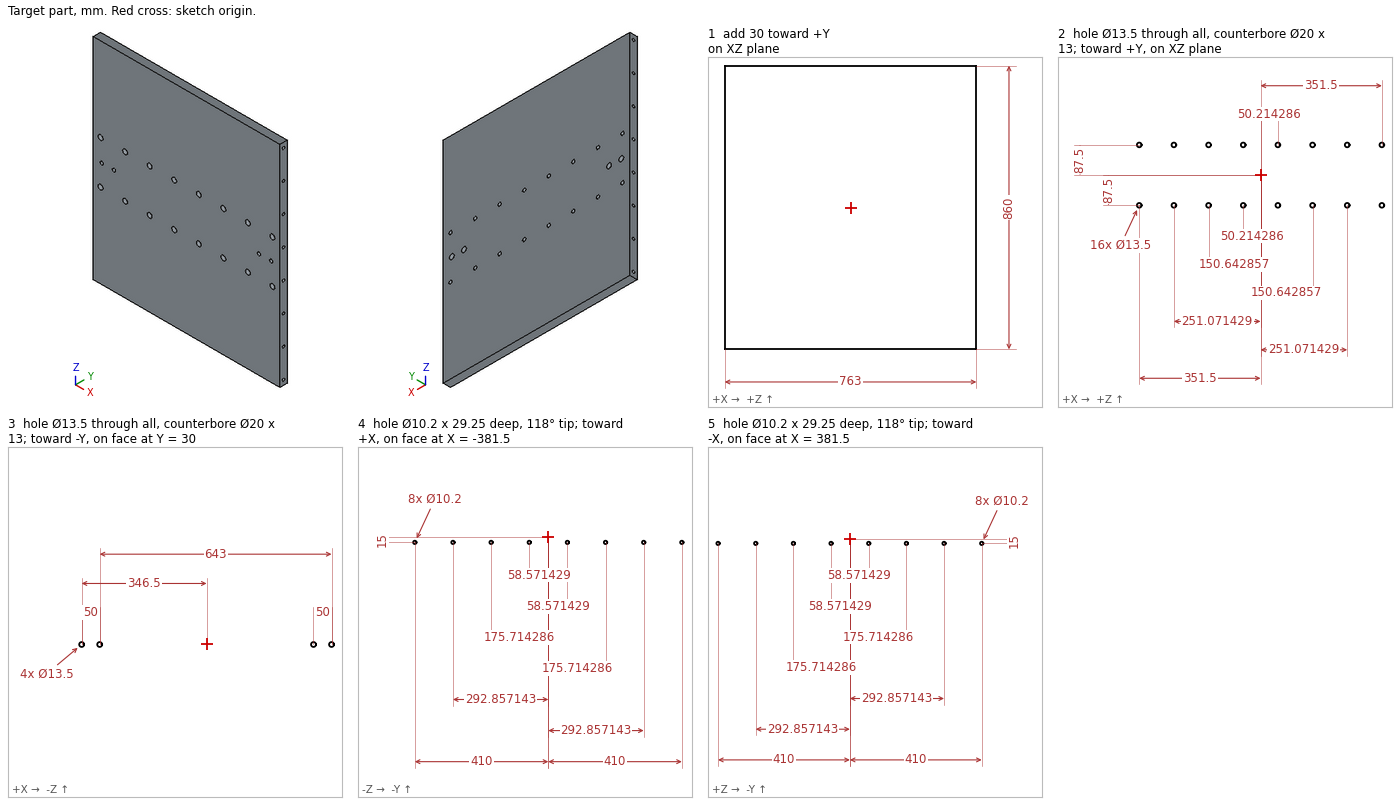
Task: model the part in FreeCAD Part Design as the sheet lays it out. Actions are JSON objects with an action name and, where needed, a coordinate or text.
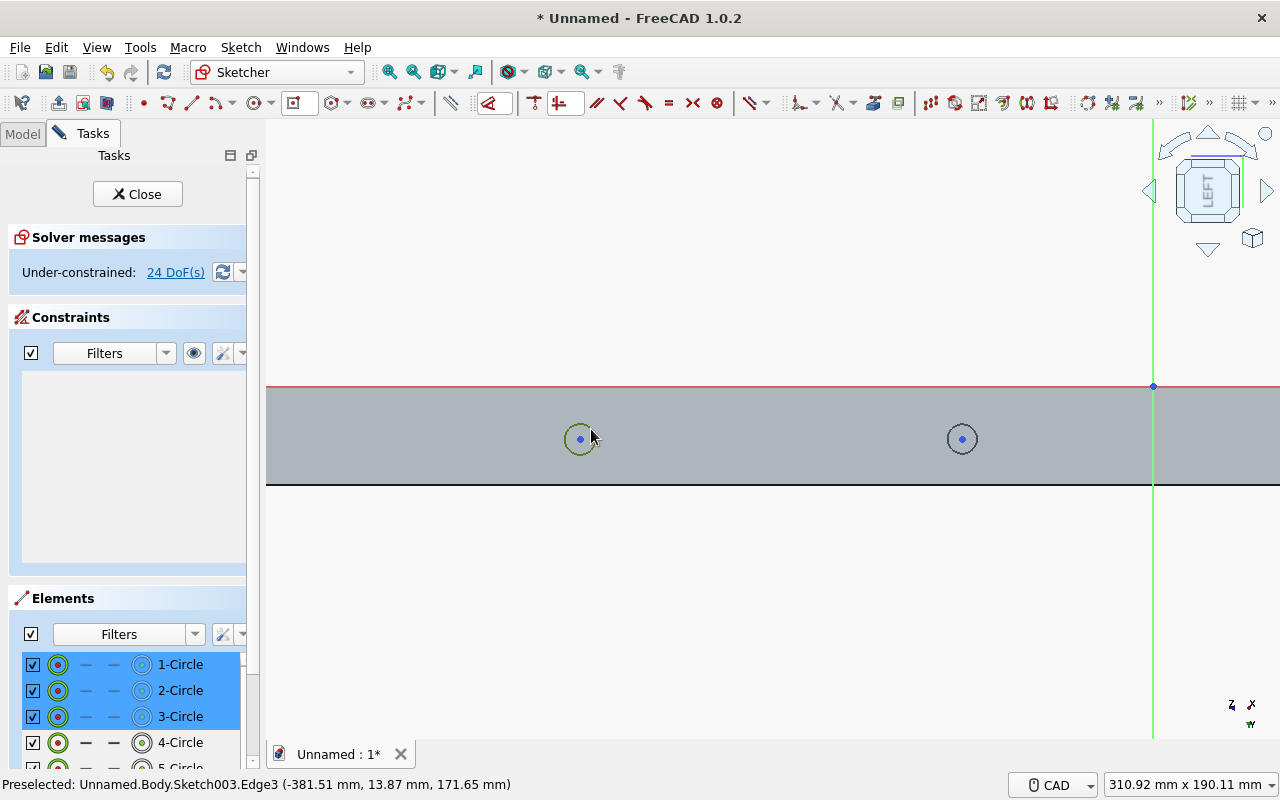
{"action": "left_click", "coordinate": [973, 429]}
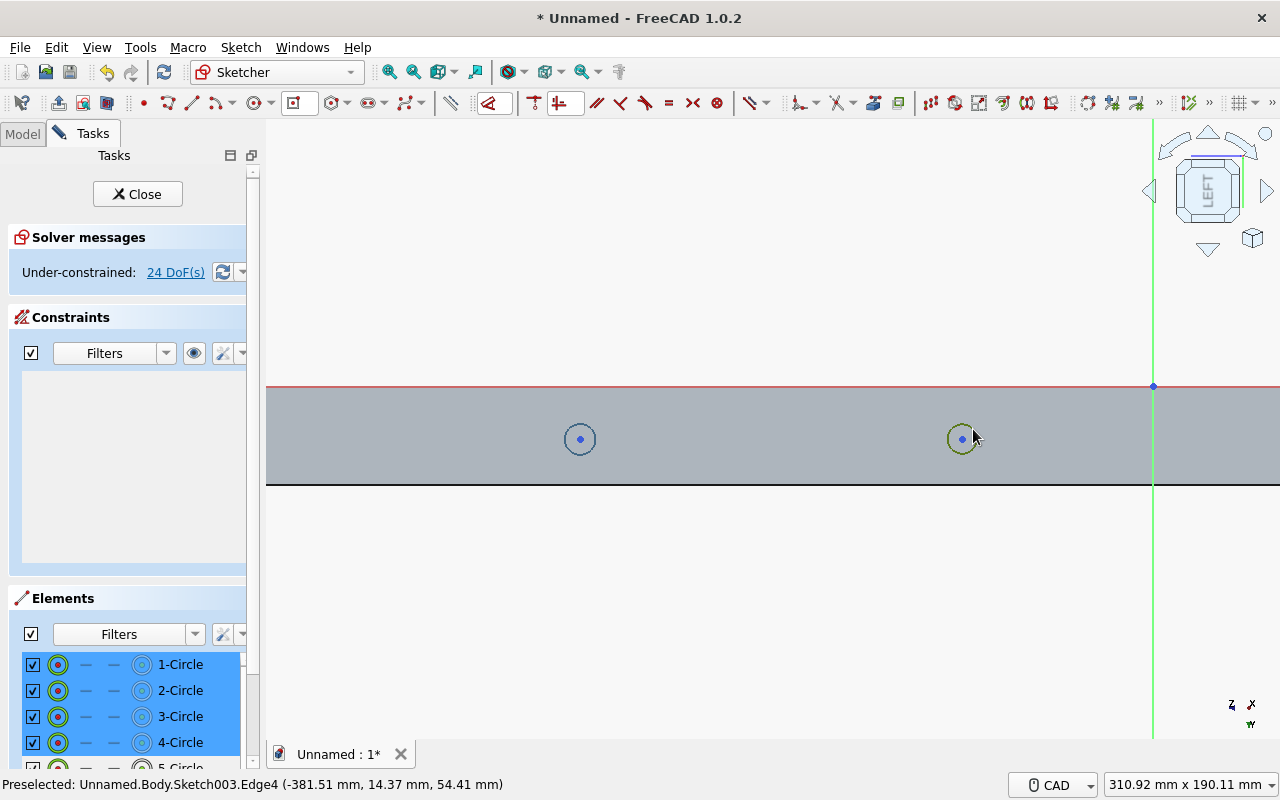
{"action": "scroll", "coordinate": [591, 431], "scroll_direction": "down", "scroll_amount": 8}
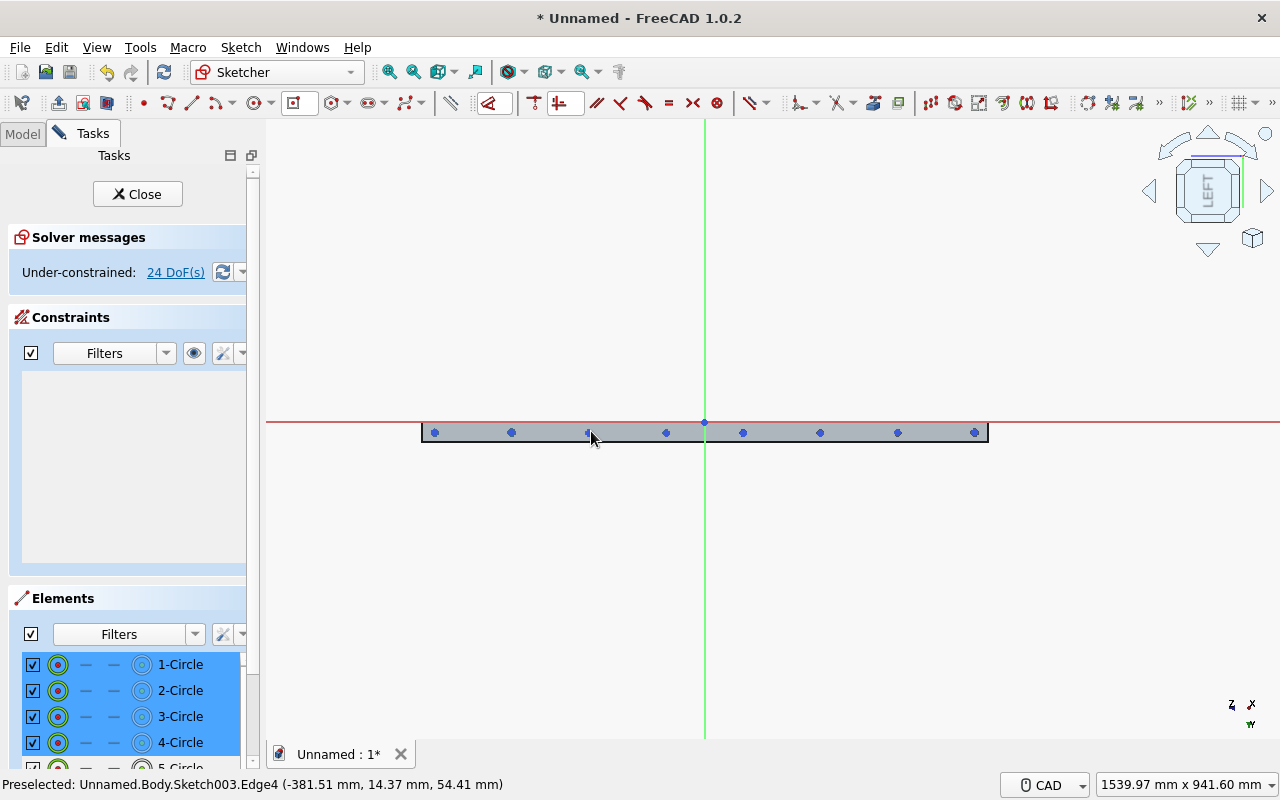
{"action": "scroll", "coordinate": [745, 431], "scroll_direction": "up", "scroll_amount": 8}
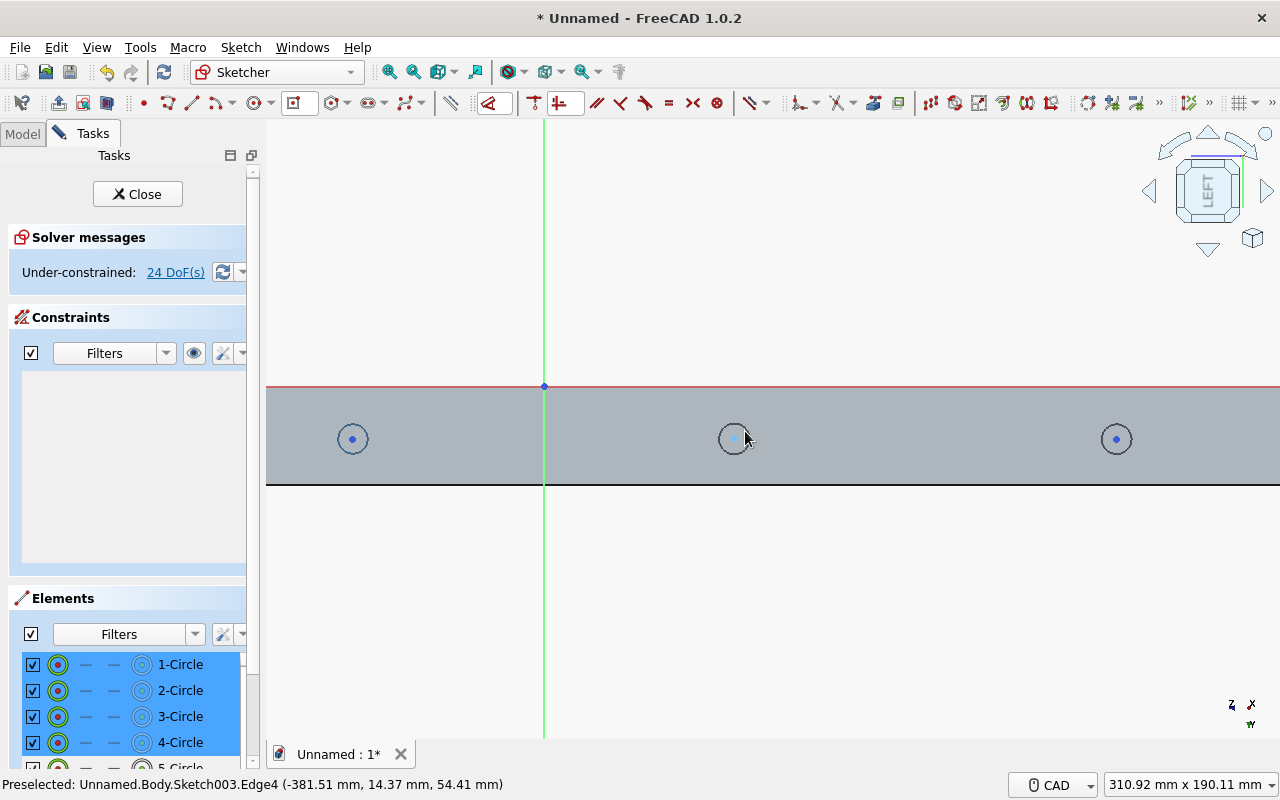
{"action": "left_click", "coordinate": [745, 428]}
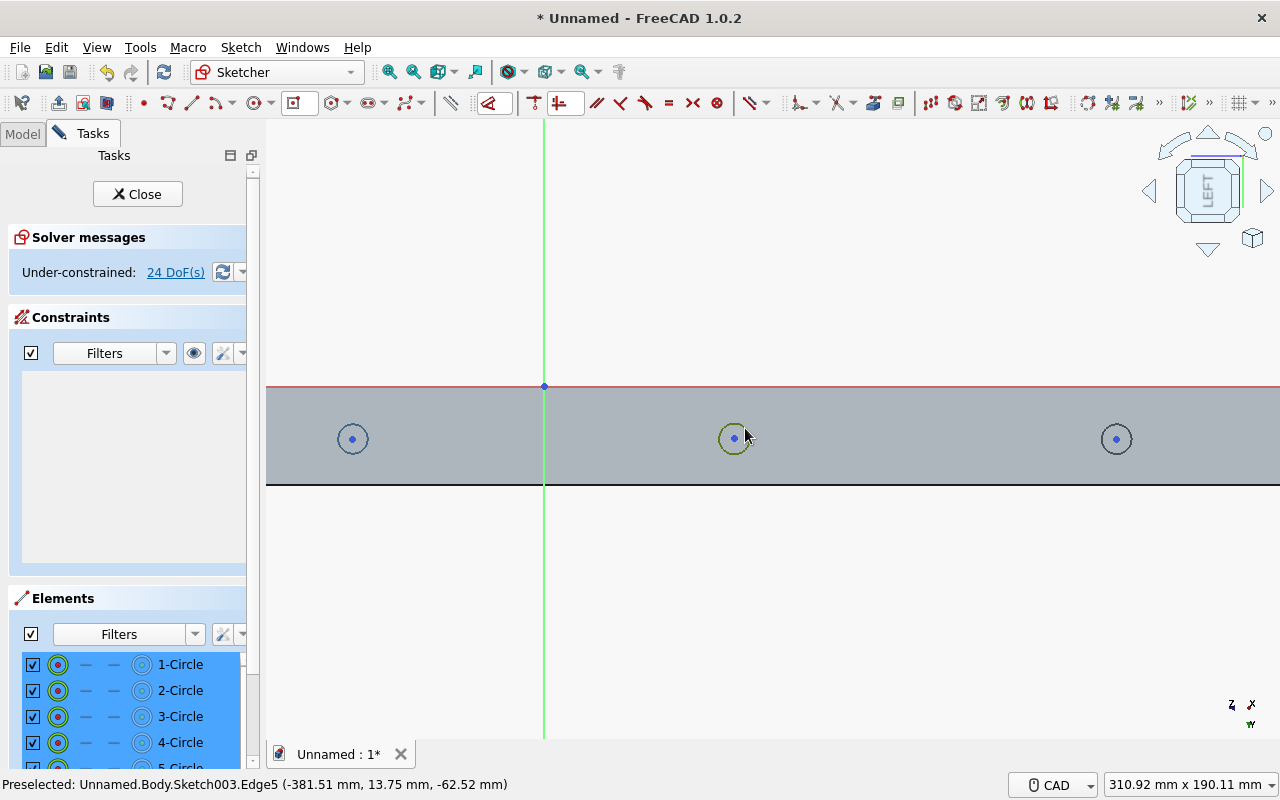
{"action": "left_click", "coordinate": [1106, 429]}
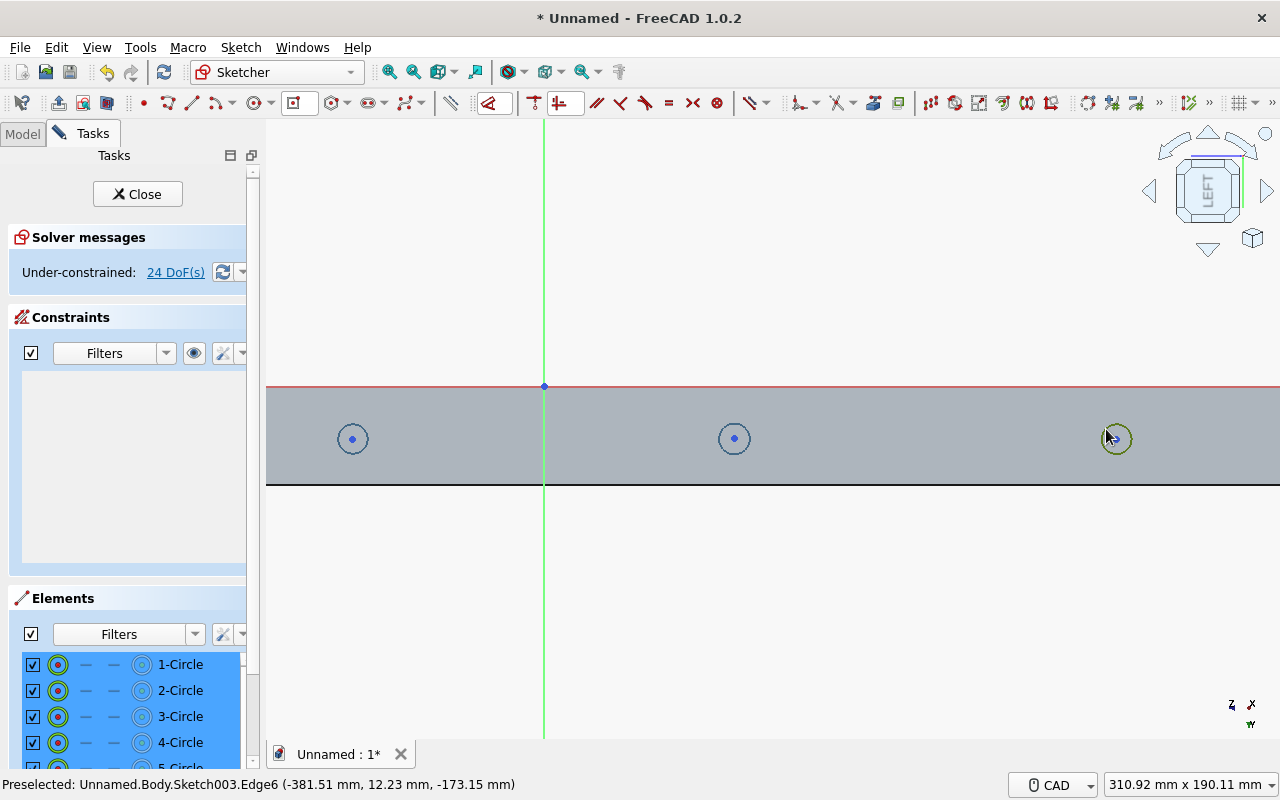
{"action": "scroll", "coordinate": [745, 431], "scroll_direction": "down", "scroll_amount": 8}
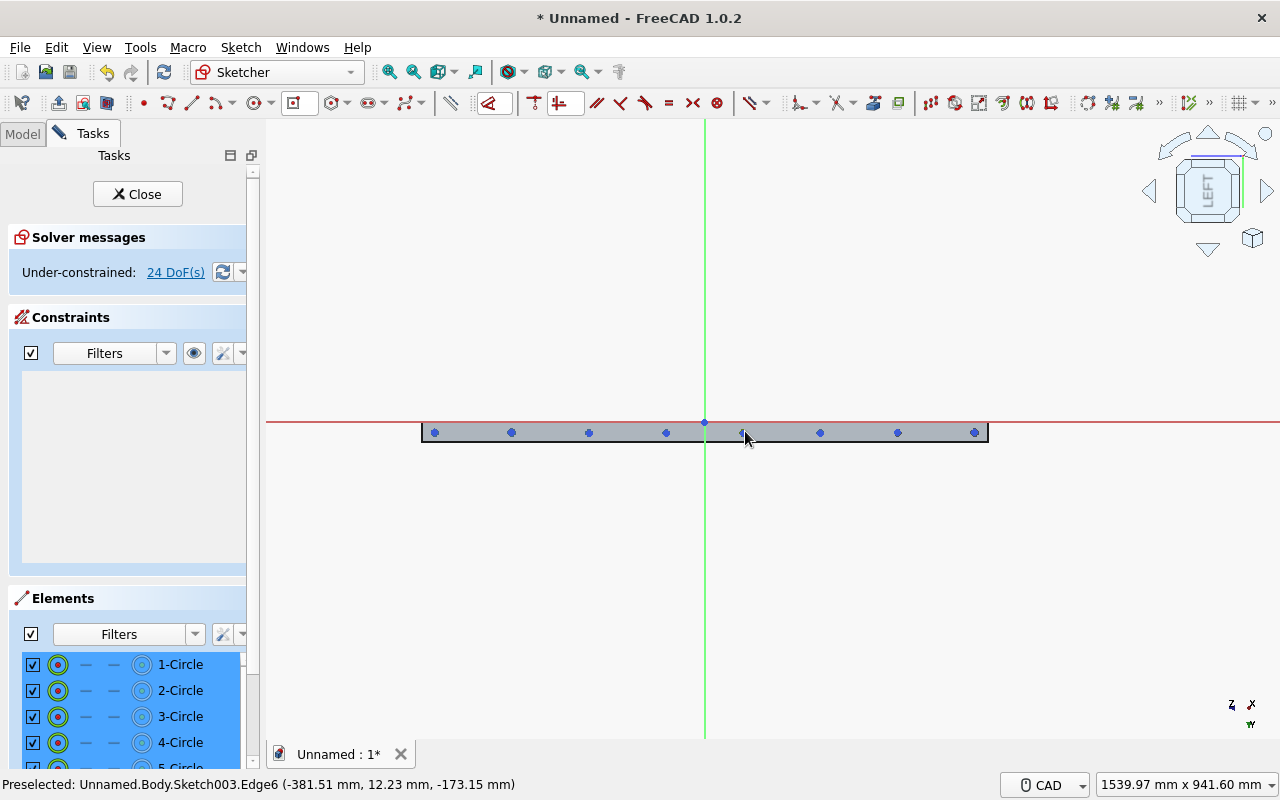
{"action": "scroll", "coordinate": [900, 431], "scroll_direction": "up", "scroll_amount": 8}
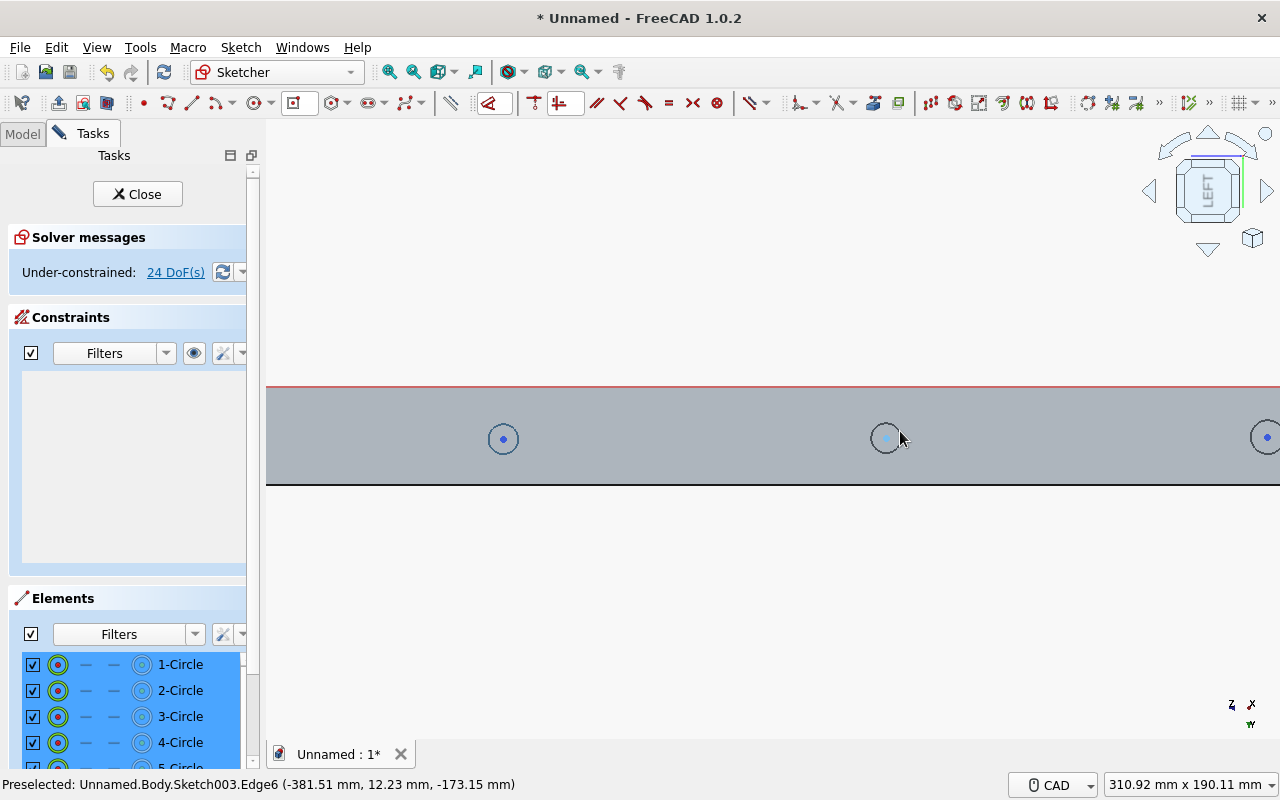
{"action": "left_click", "coordinate": [897, 428]}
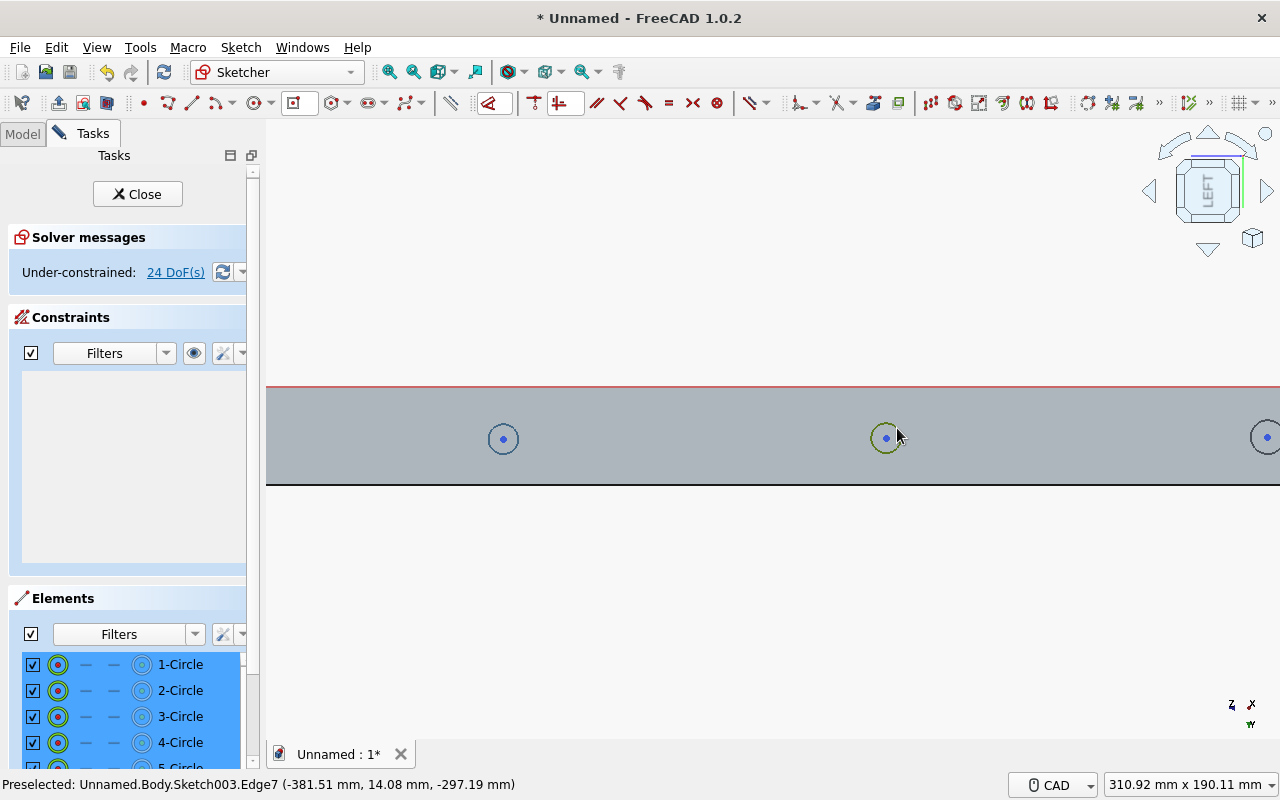
{"action": "scroll", "coordinate": [900, 431], "scroll_direction": "down", "scroll_amount": 8}